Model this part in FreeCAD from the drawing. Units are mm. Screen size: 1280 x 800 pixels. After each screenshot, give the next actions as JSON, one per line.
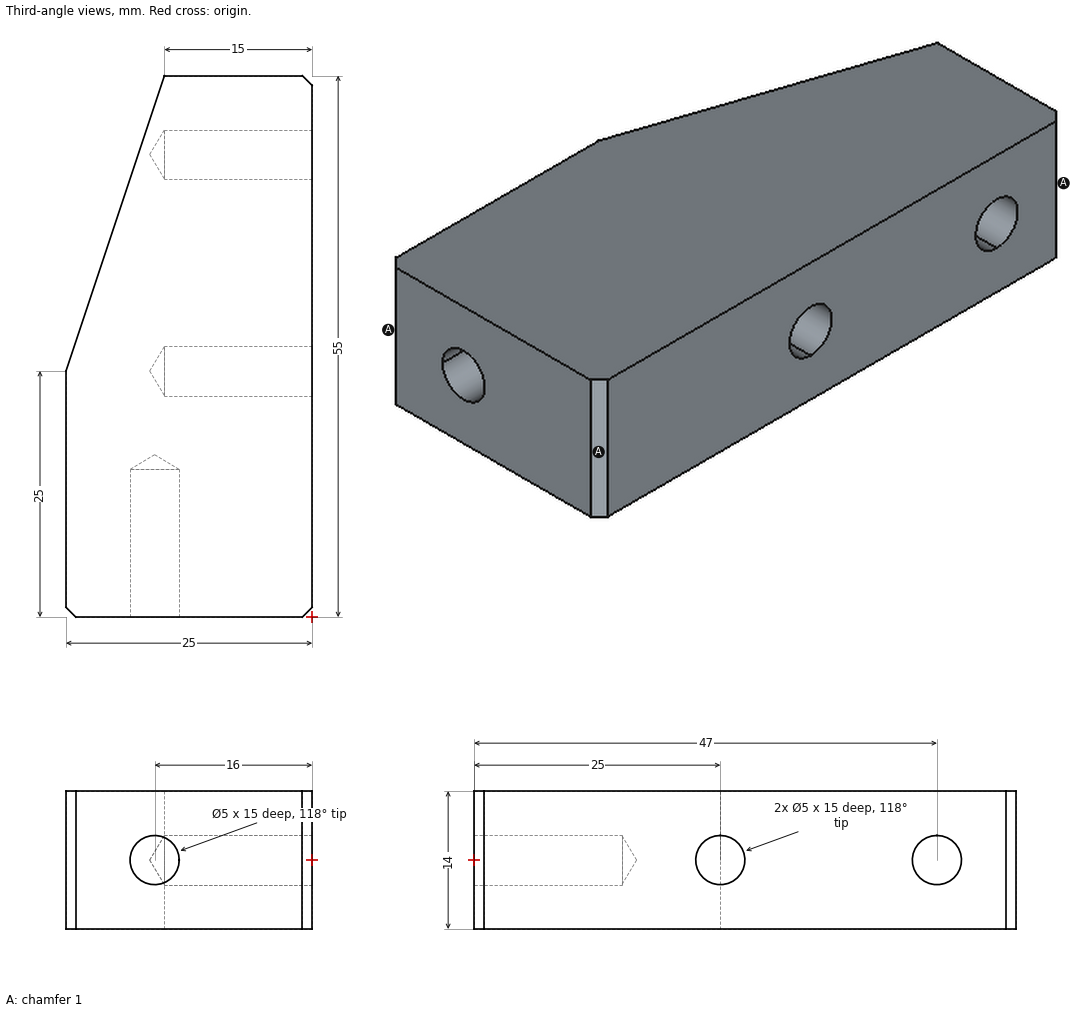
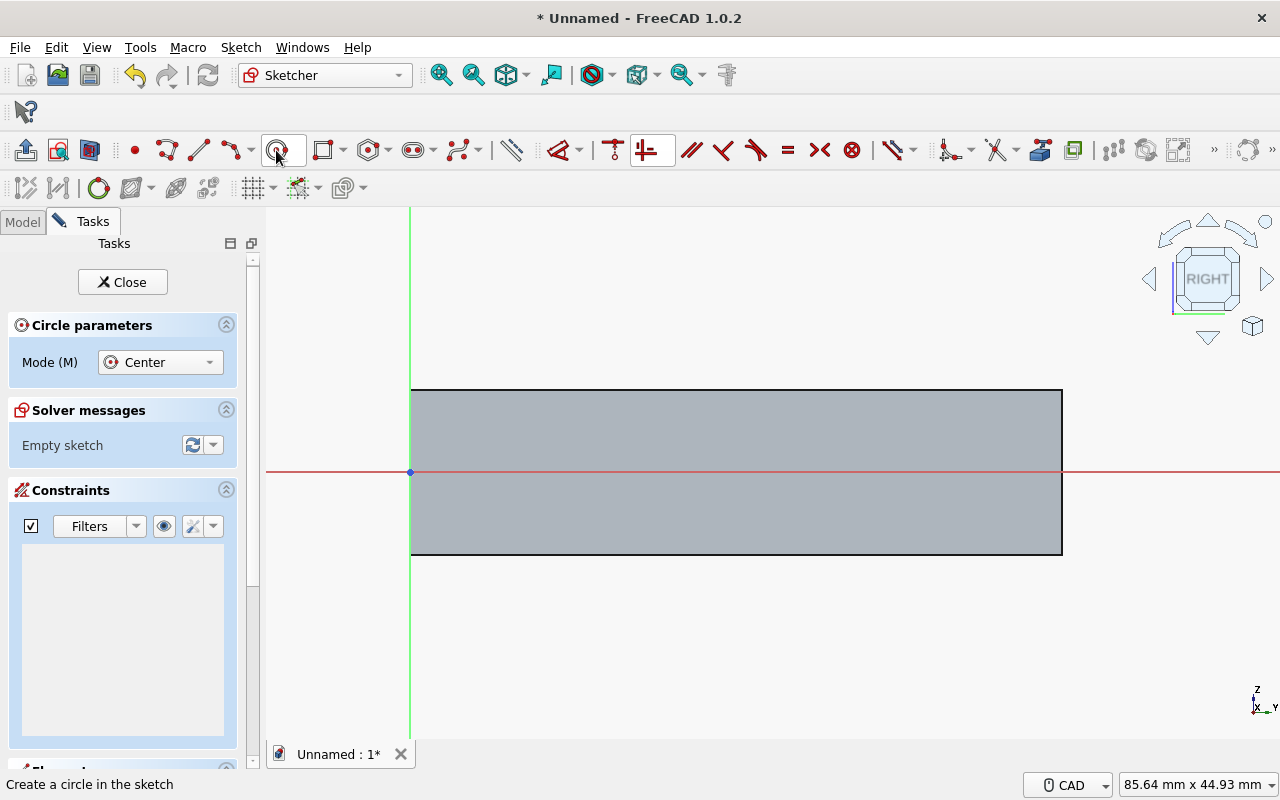
{"action": "left_click", "coordinate": [706, 472]}
{"action": "mouse_move", "coordinate": [727, 451]}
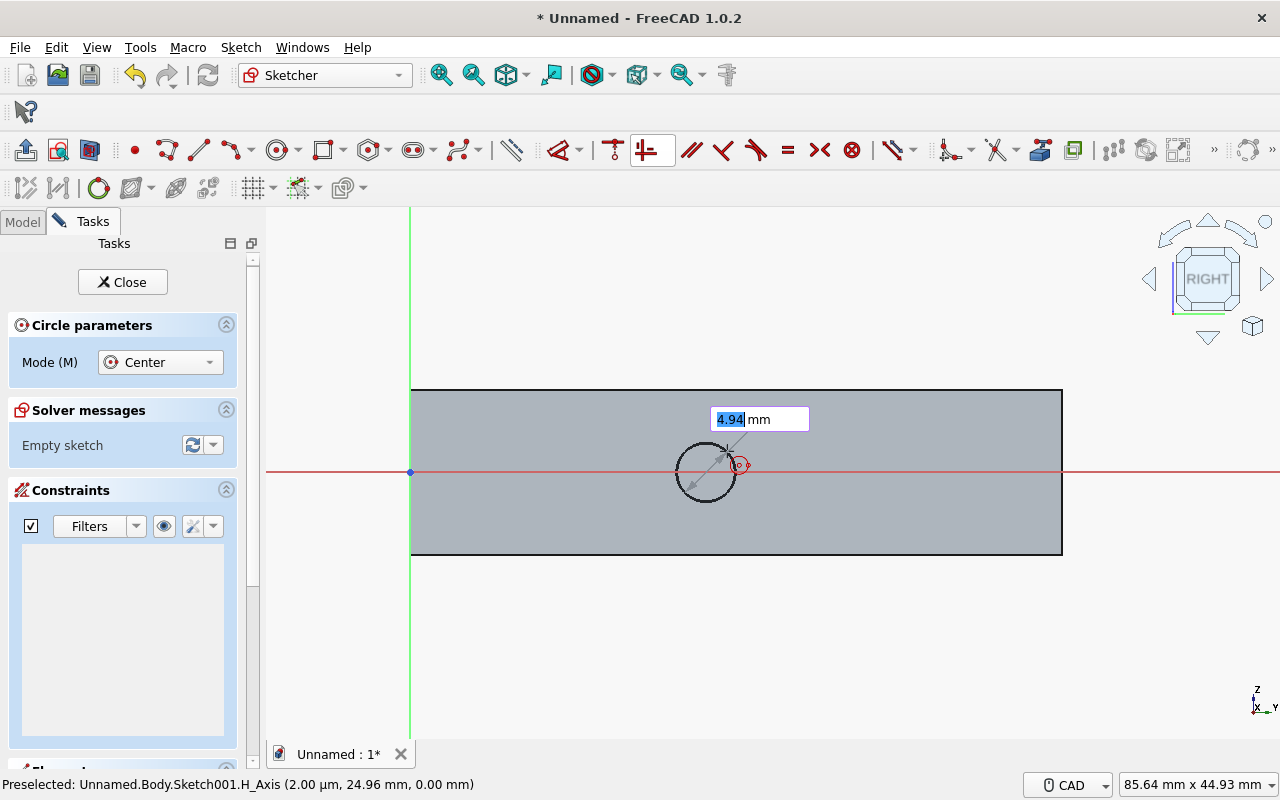
{"action": "type", "text": "5"}
{"action": "key", "text": "Return"}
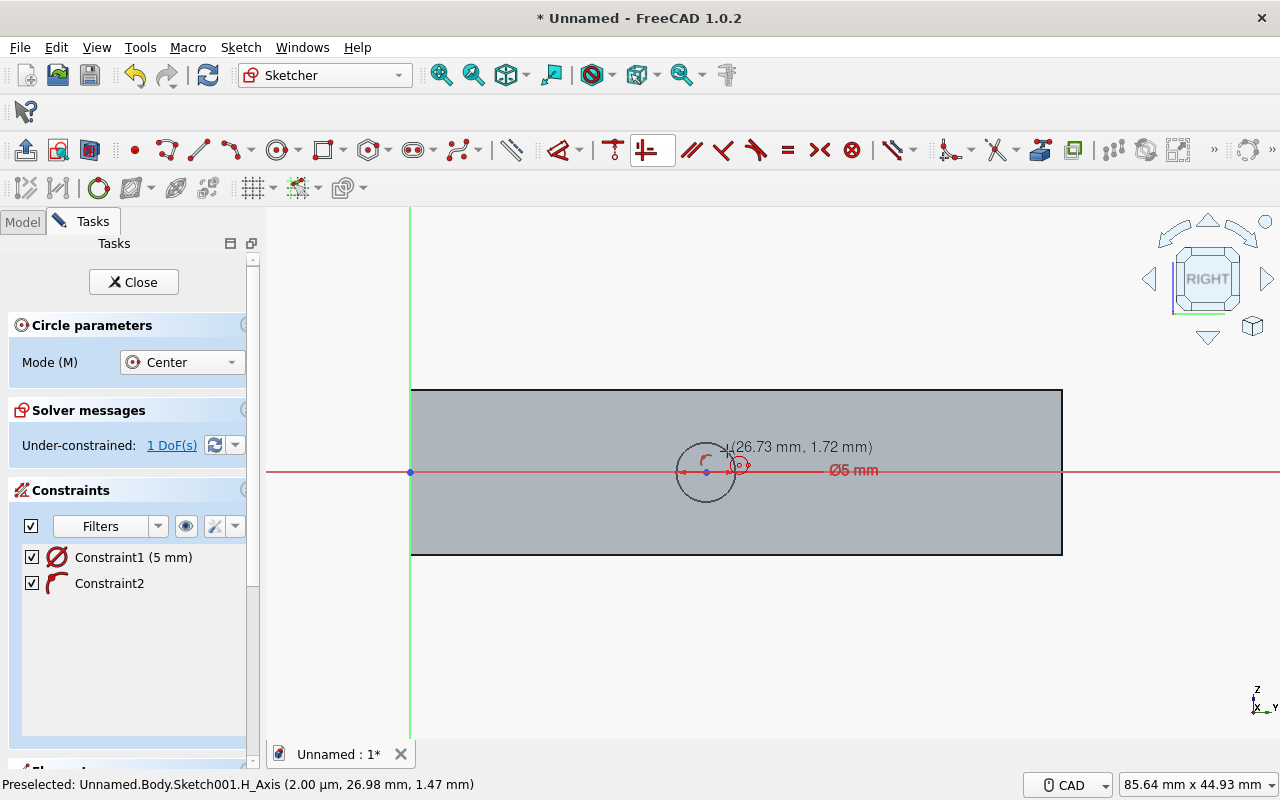
{"action": "left_click", "coordinate": [967, 472]}
{"action": "mouse_move", "coordinate": [988, 451]}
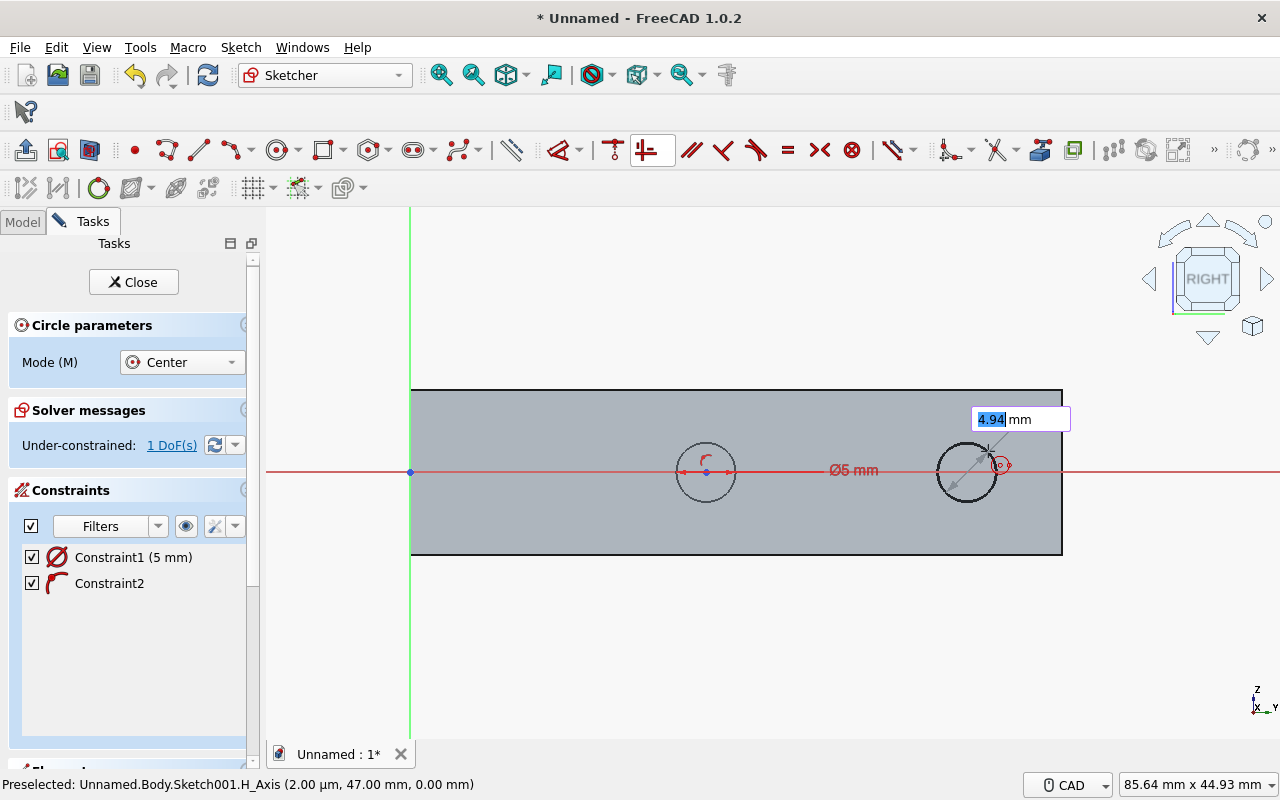
{"action": "type", "text": "5"}
{"action": "key", "text": "Return"}
{"action": "key", "text": "Escape"}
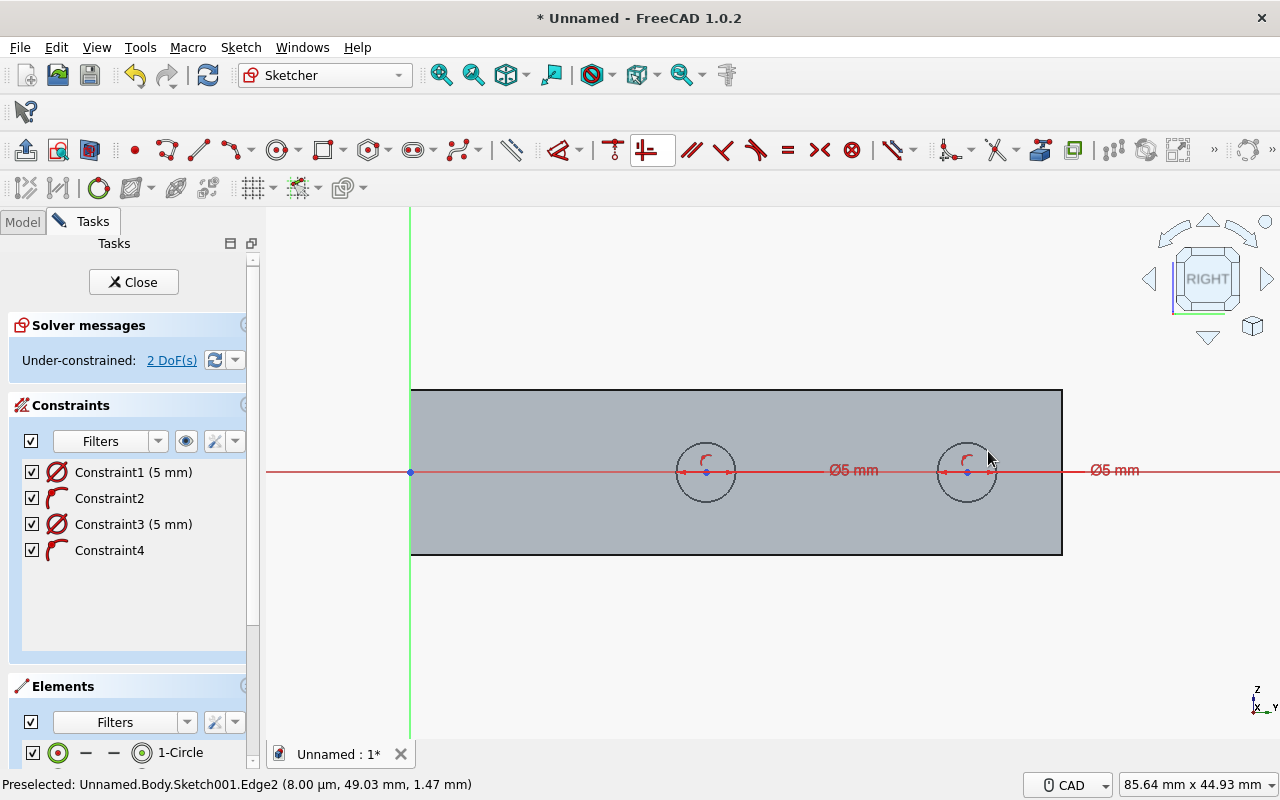
{"action": "left_click", "coordinate": [558, 150]}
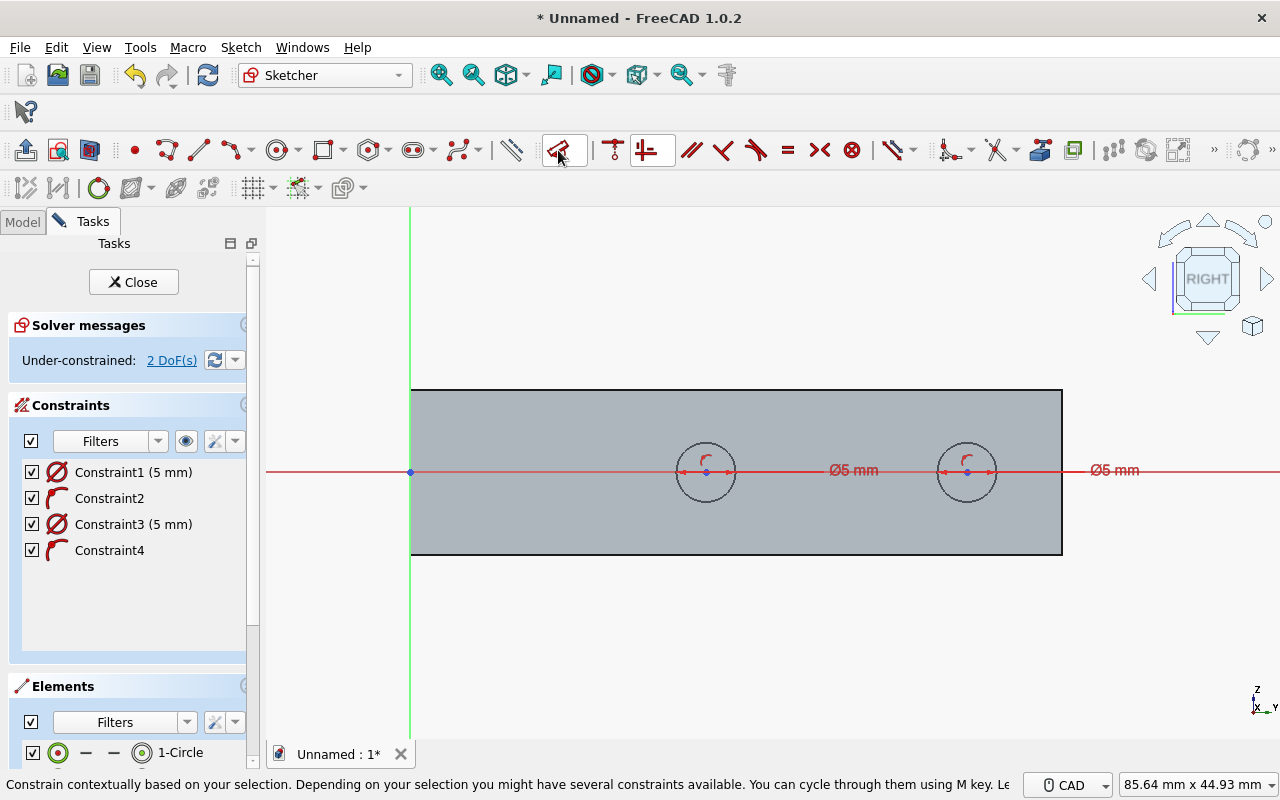
{"action": "left_click", "coordinate": [706, 472]}
{"action": "left_click", "coordinate": [558, 506]}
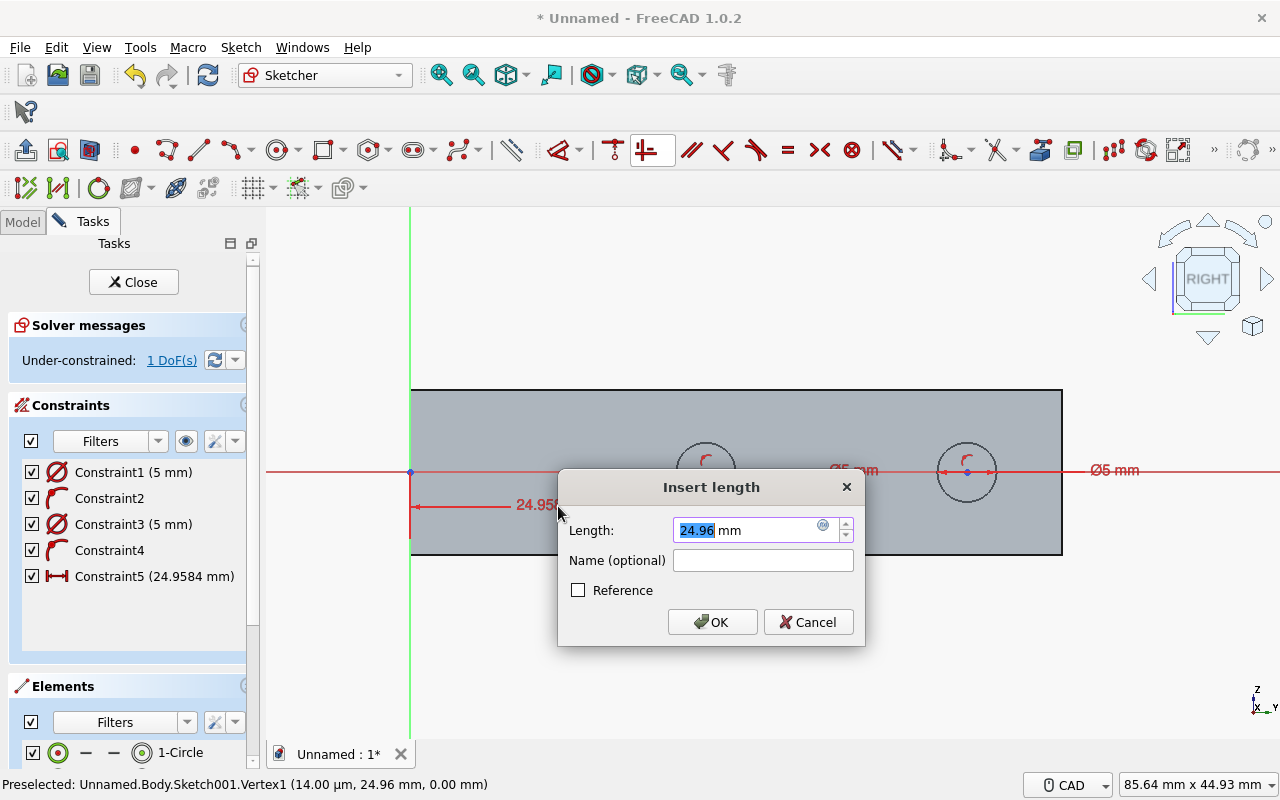
{"action": "type", "text": "25"}
{"action": "key", "text": "Return"}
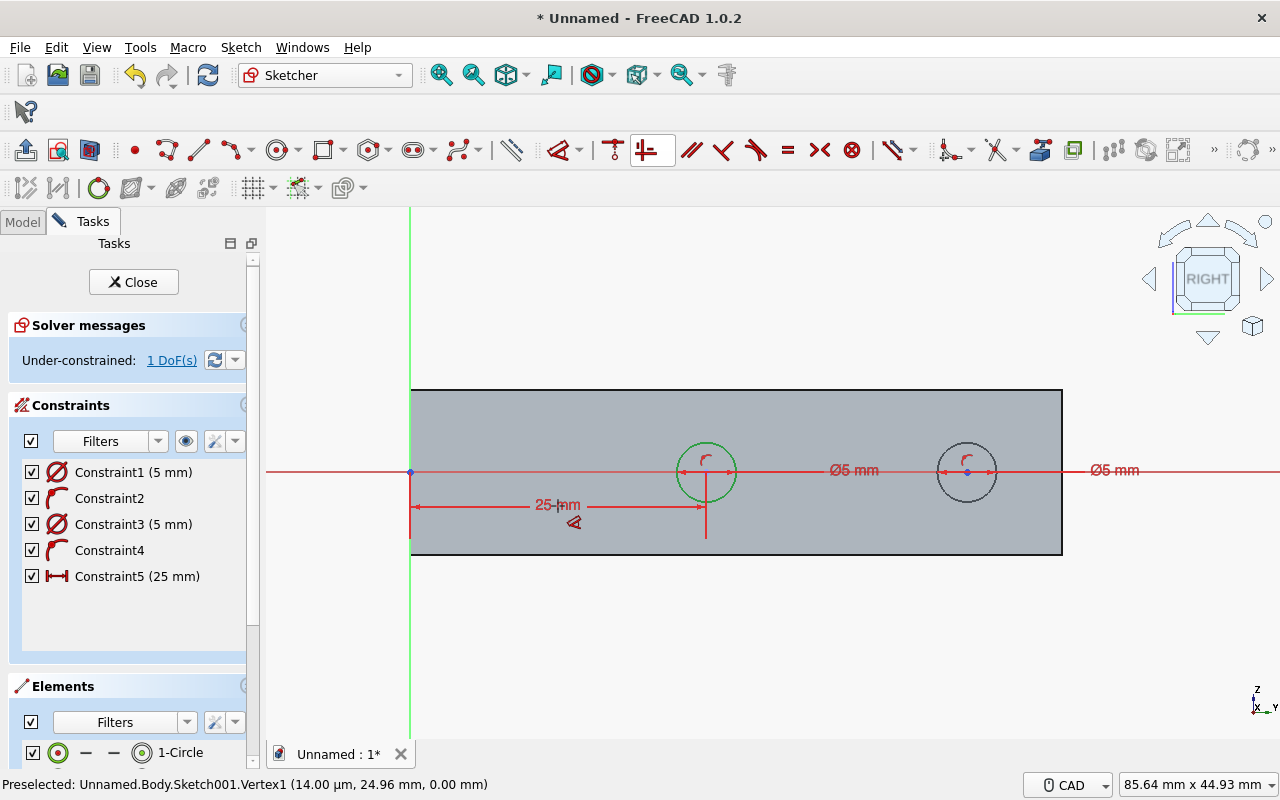
{"action": "left_click", "coordinate": [967, 472]}
{"action": "left_click", "coordinate": [817, 506]}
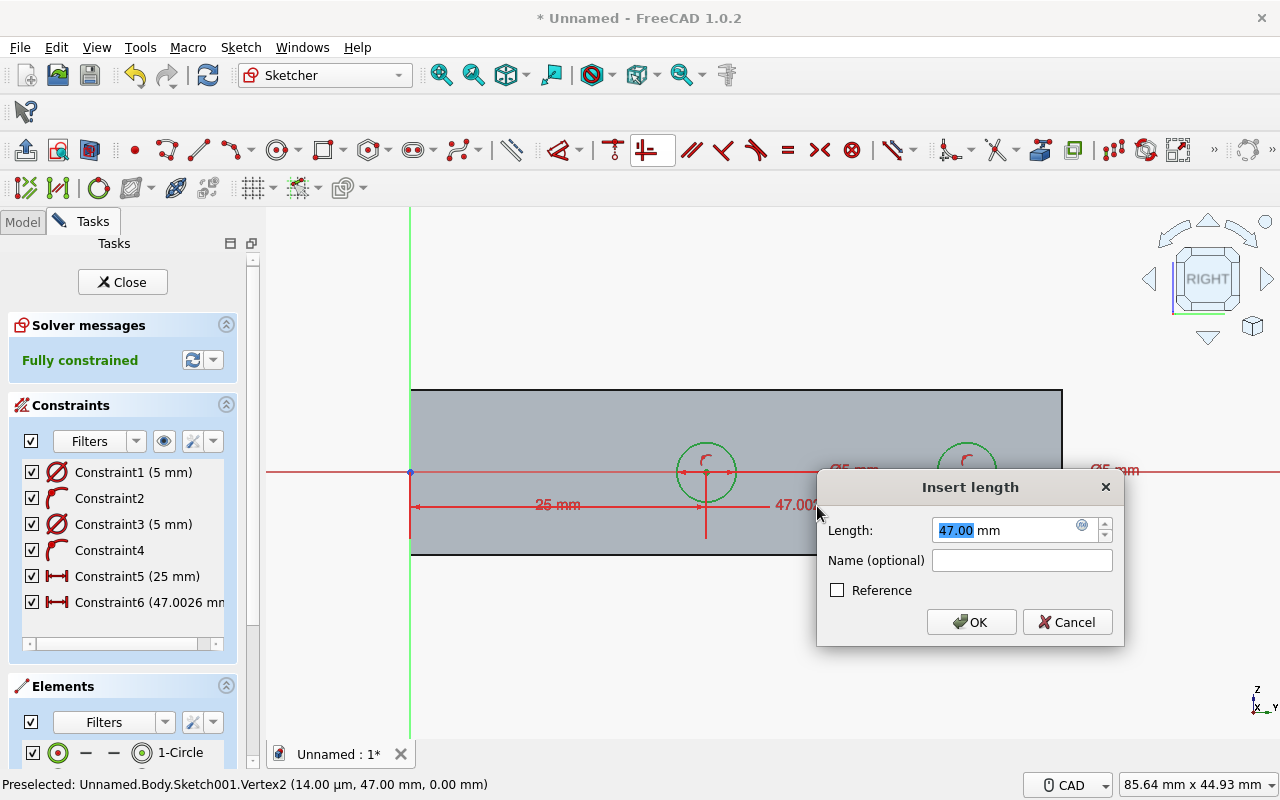
{"action": "type", "text": "47"}
{"action": "key", "text": "Return"}
{"action": "key", "text": "Escape"}